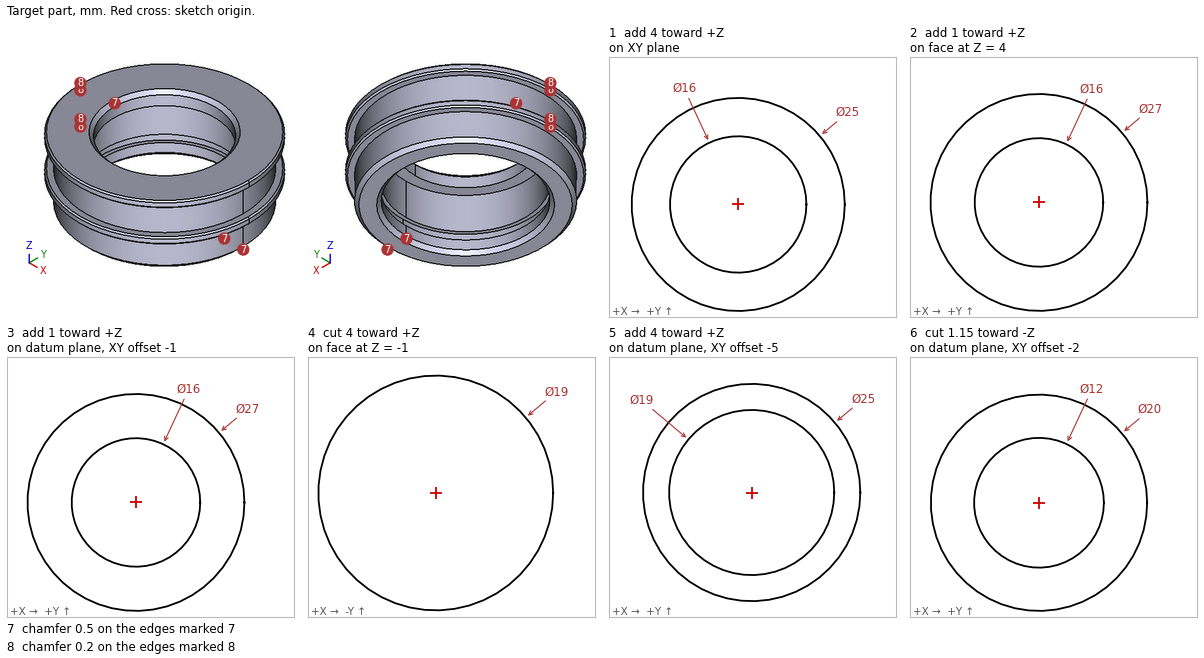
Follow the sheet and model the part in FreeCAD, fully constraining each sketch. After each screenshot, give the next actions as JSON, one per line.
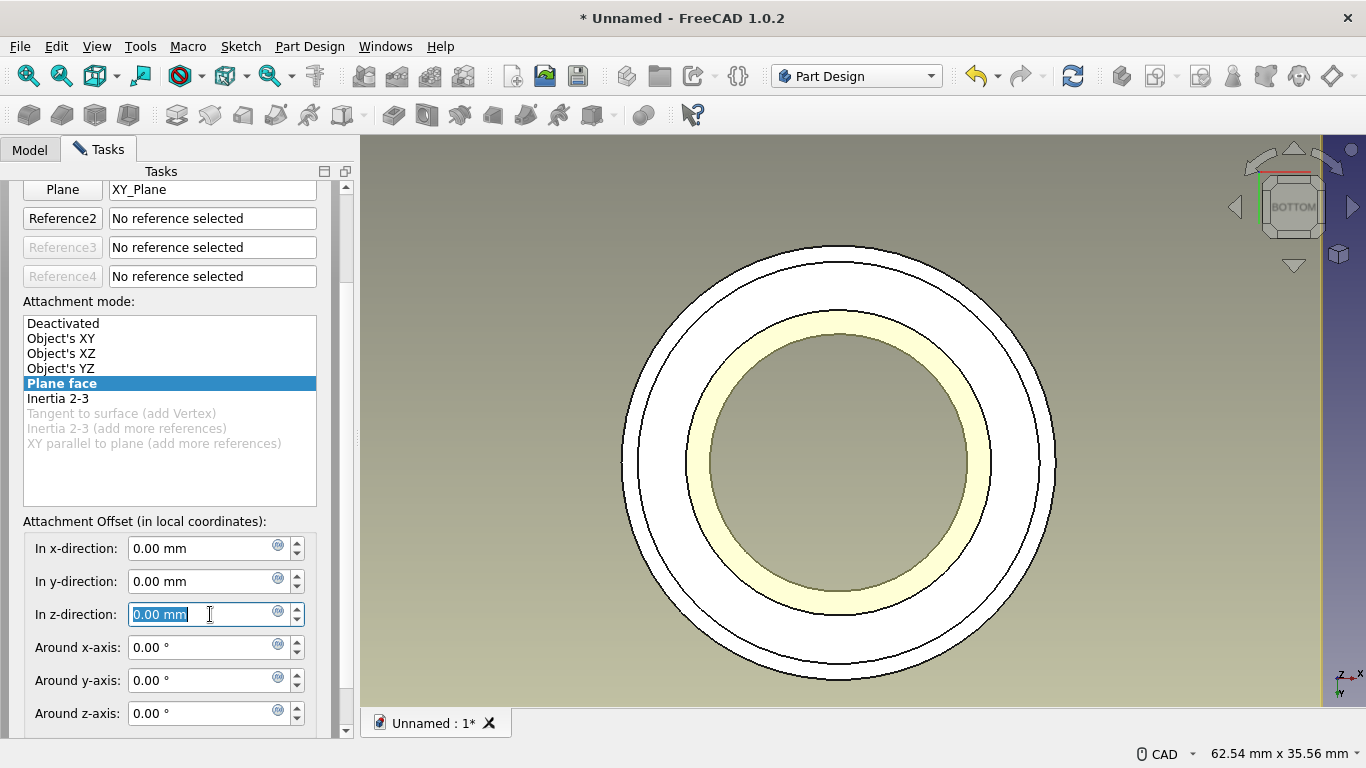
{"action": "type", "text": "-2"}
{"action": "key", "text": "Tab"}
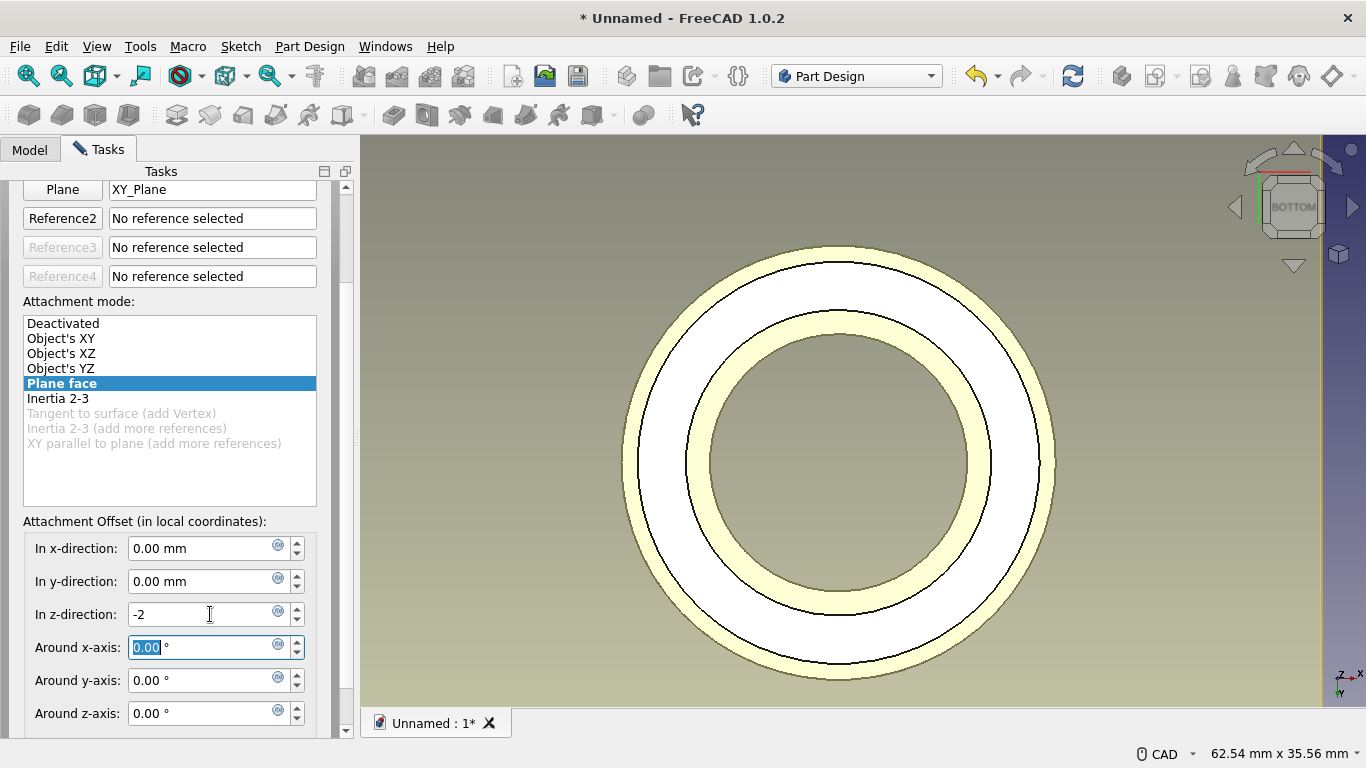
{"action": "scroll", "coordinate": [346, 460], "scroll_direction": "up", "scroll_amount": 3}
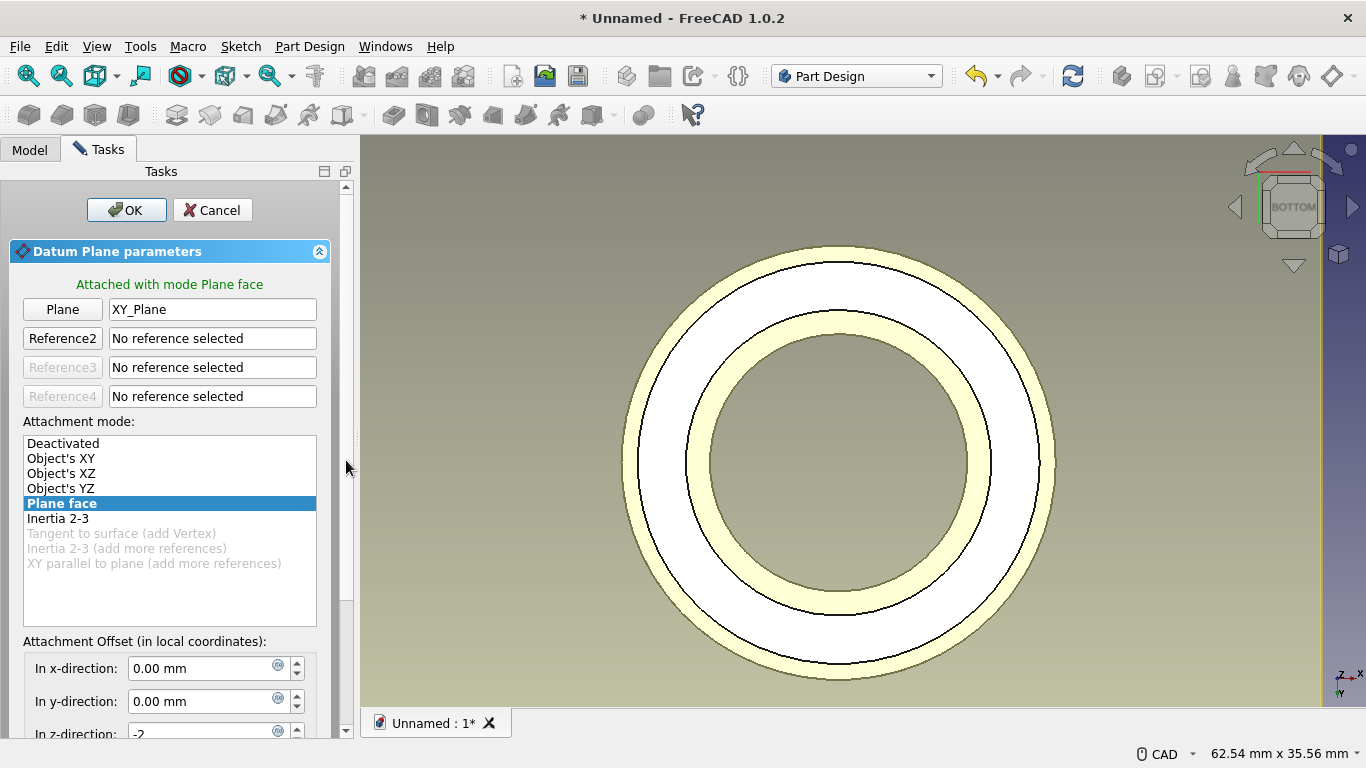
{"action": "left_click", "coordinate": [127, 210]}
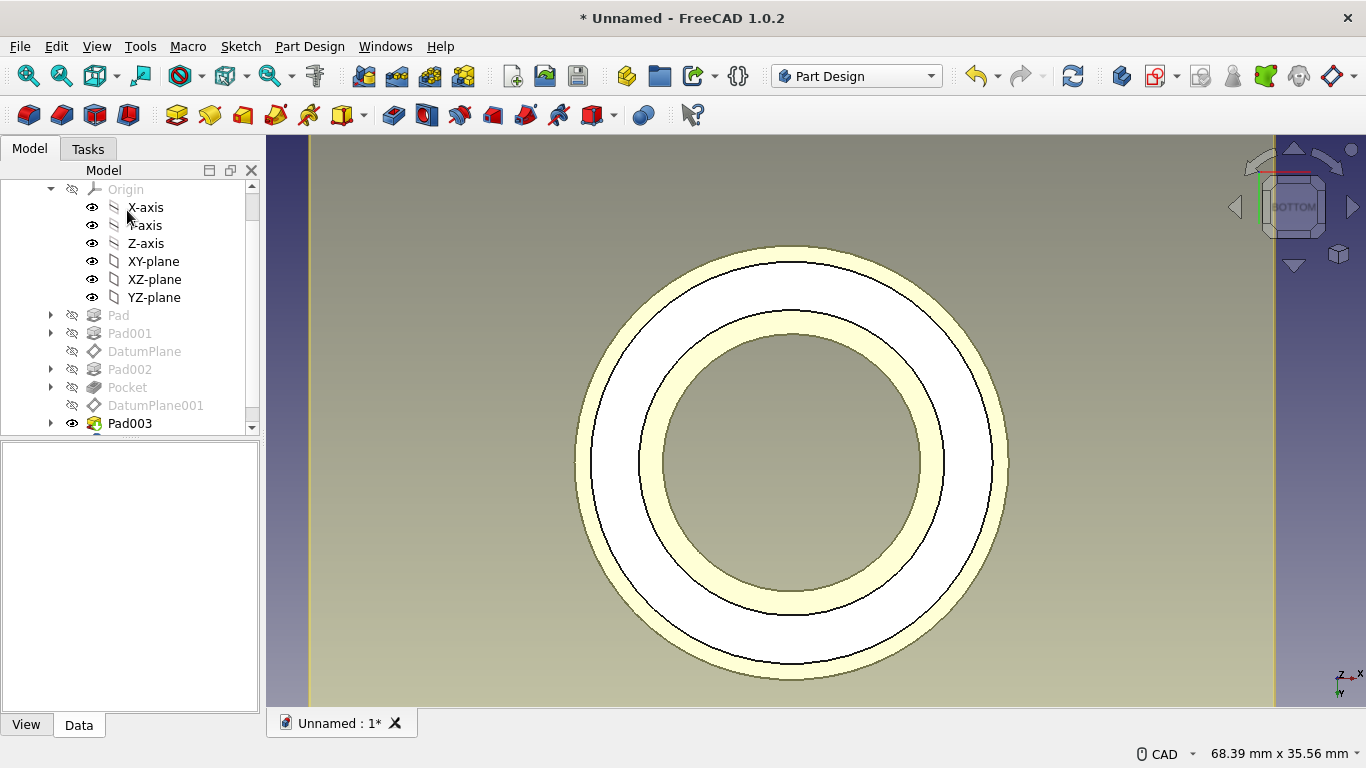
{"action": "scroll", "coordinate": [141, 311], "scroll_direction": "down", "scroll_amount": 3}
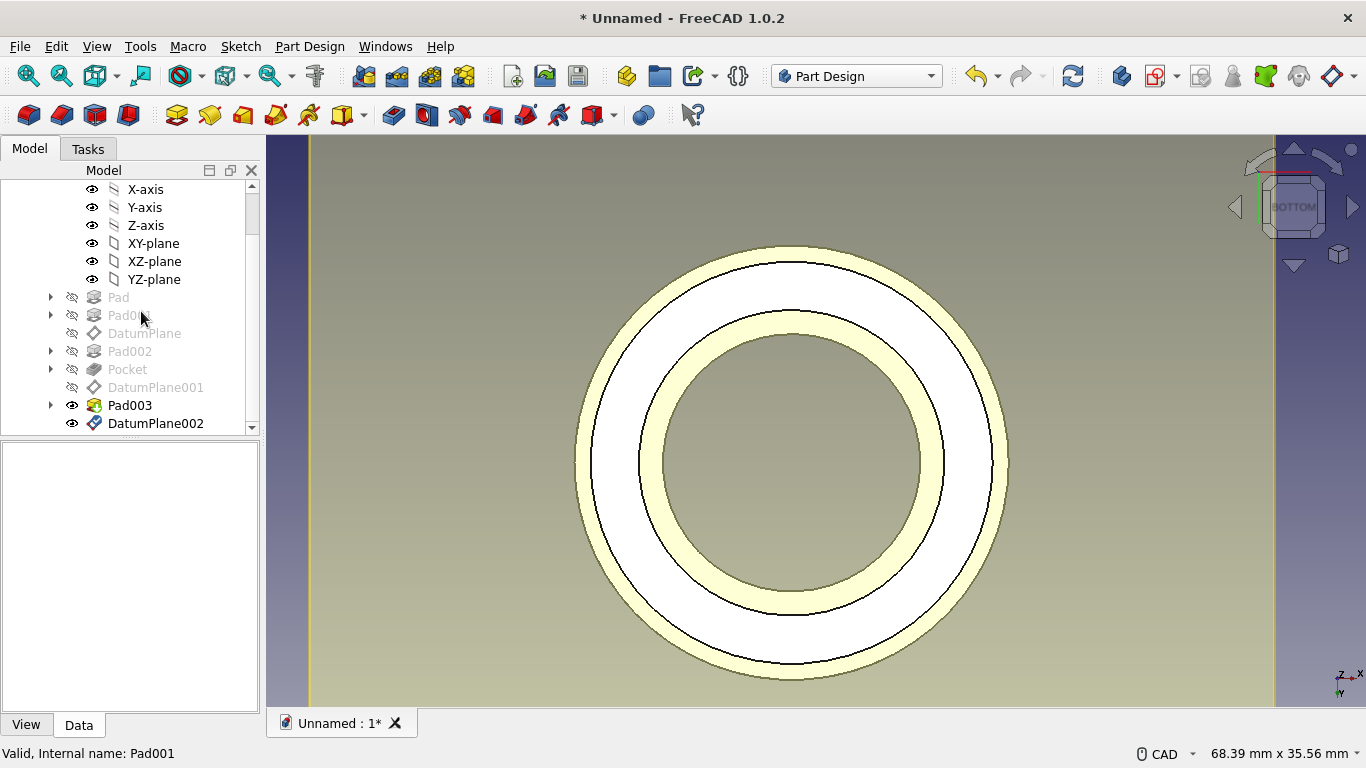
{"action": "left_click", "coordinate": [117, 423]}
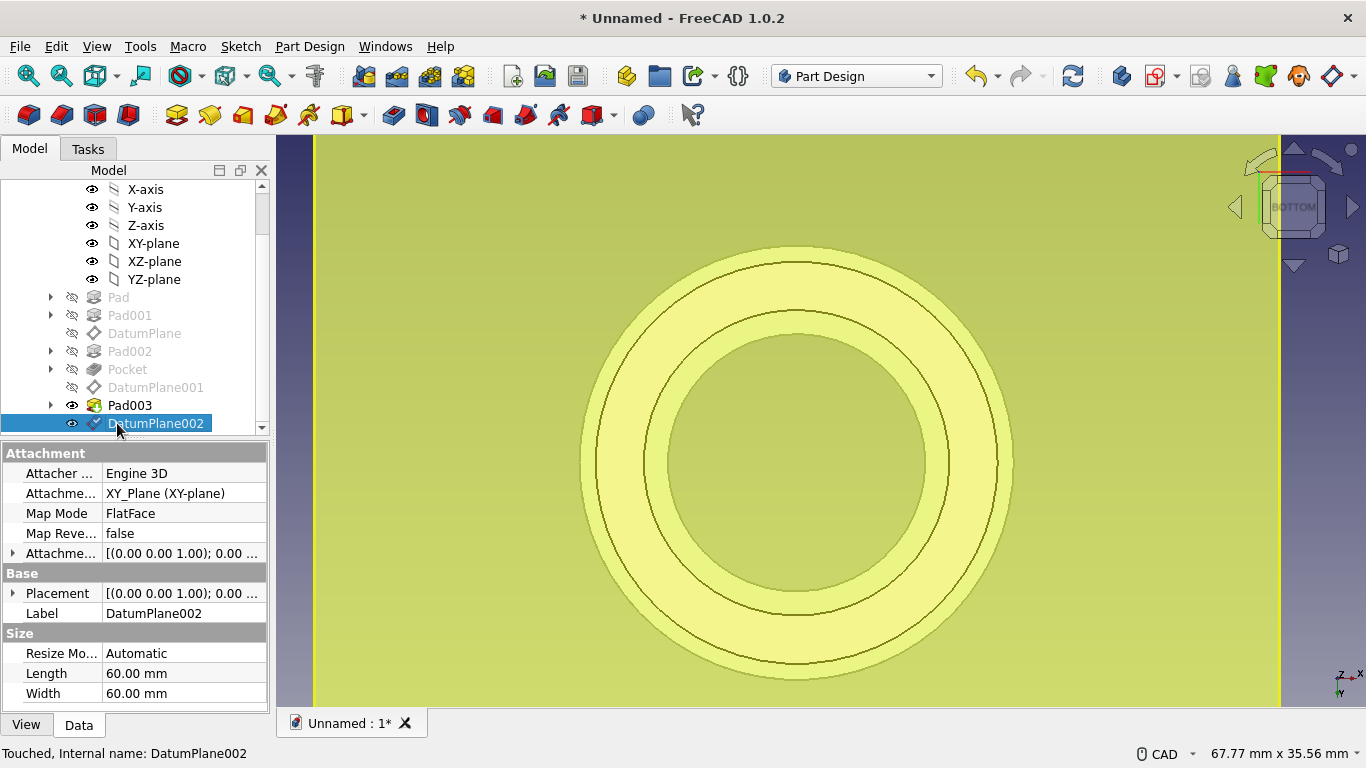
{"action": "left_click", "coordinate": [1154, 76]}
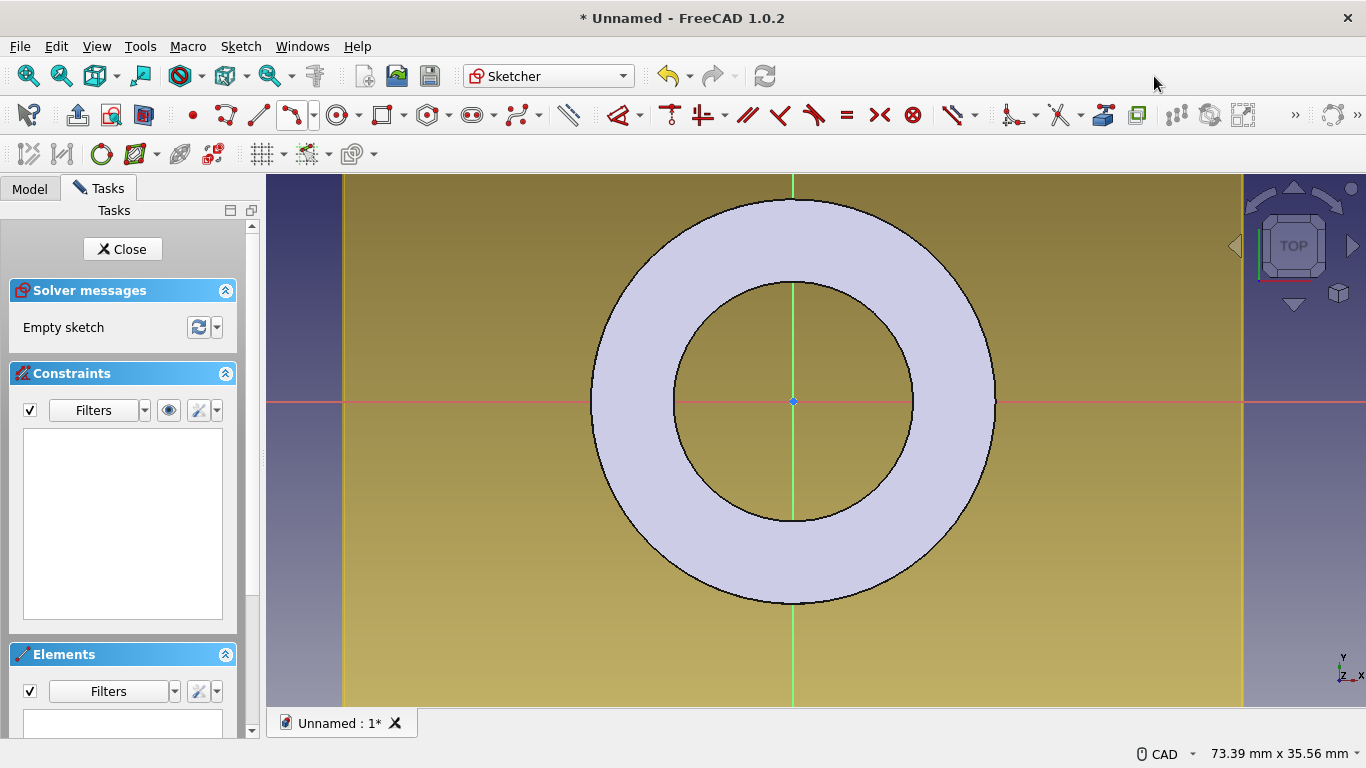
{"action": "left_click", "coordinate": [144, 116]}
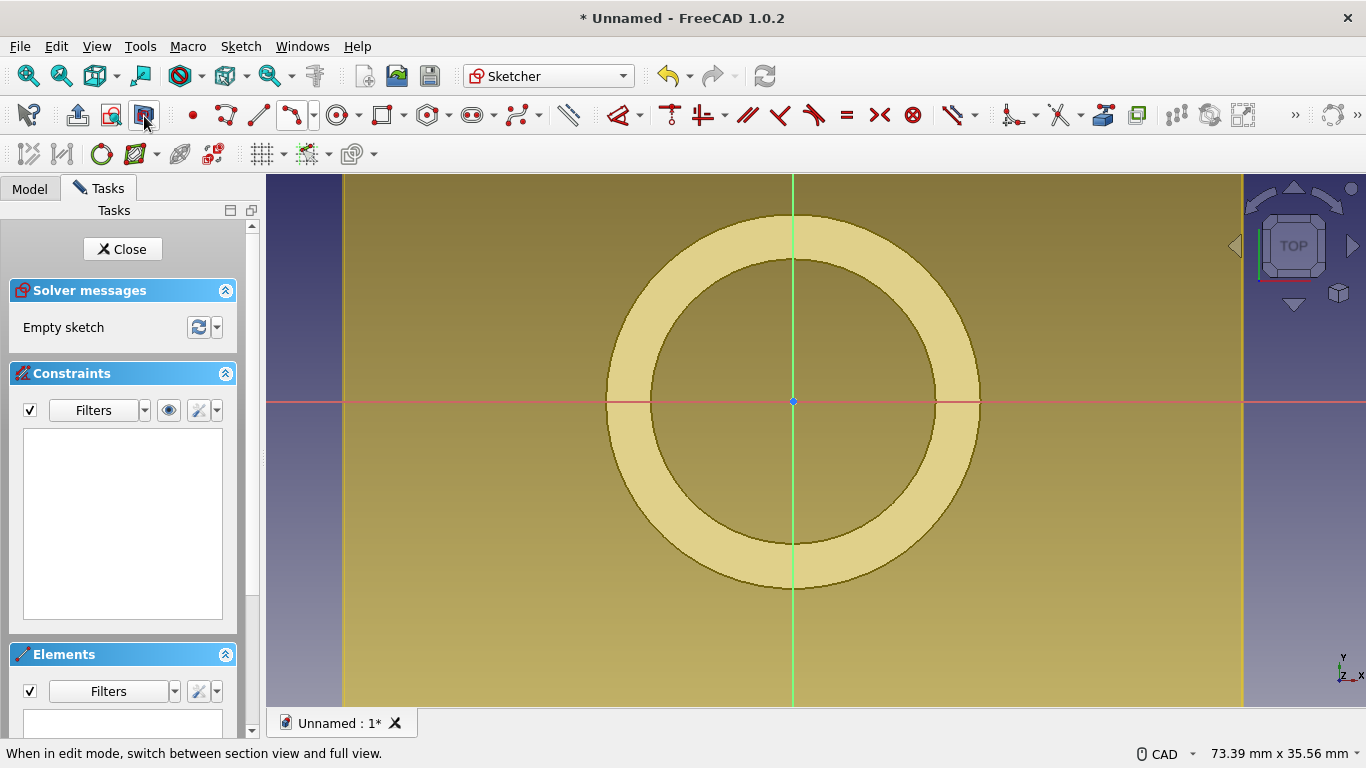
{"action": "left_click", "coordinate": [336, 116]}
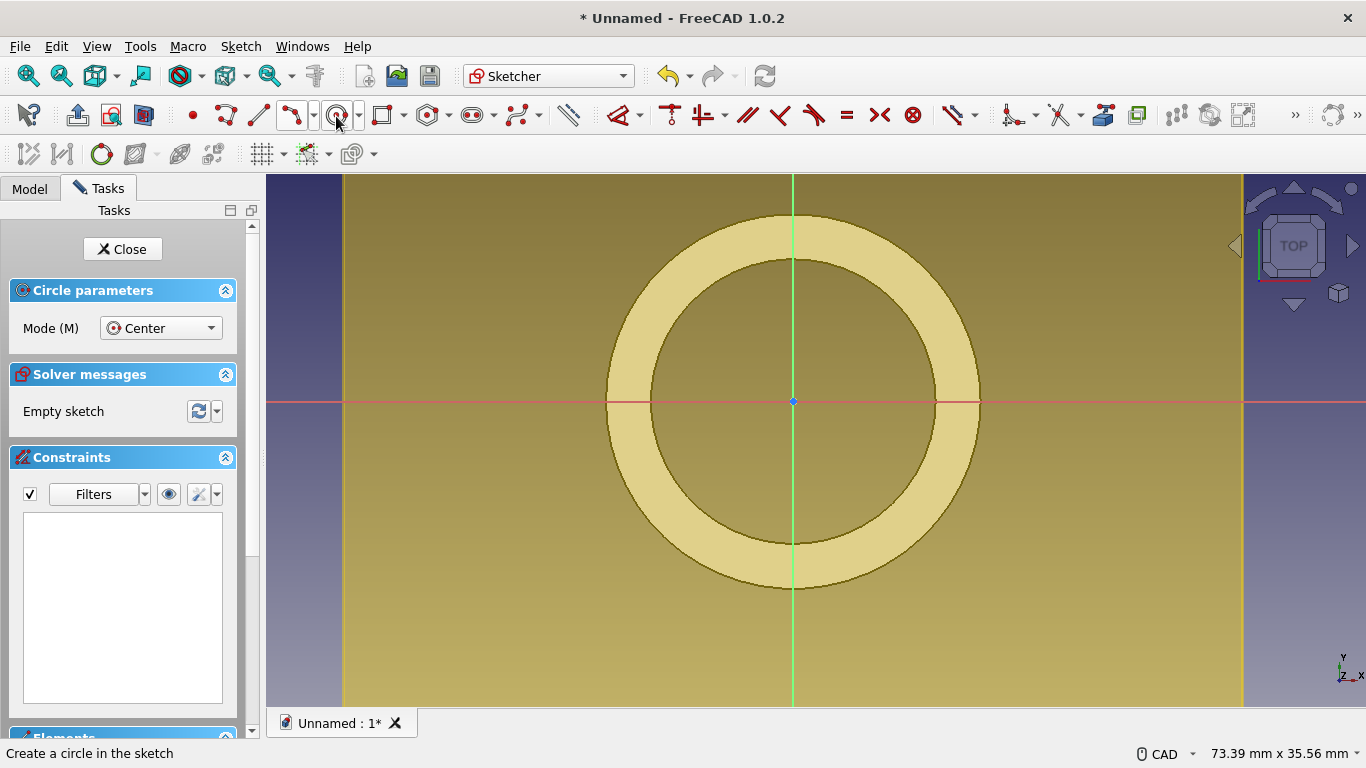
{"action": "left_click", "coordinate": [793, 402]}
{"action": "left_click", "coordinate": [899, 296]}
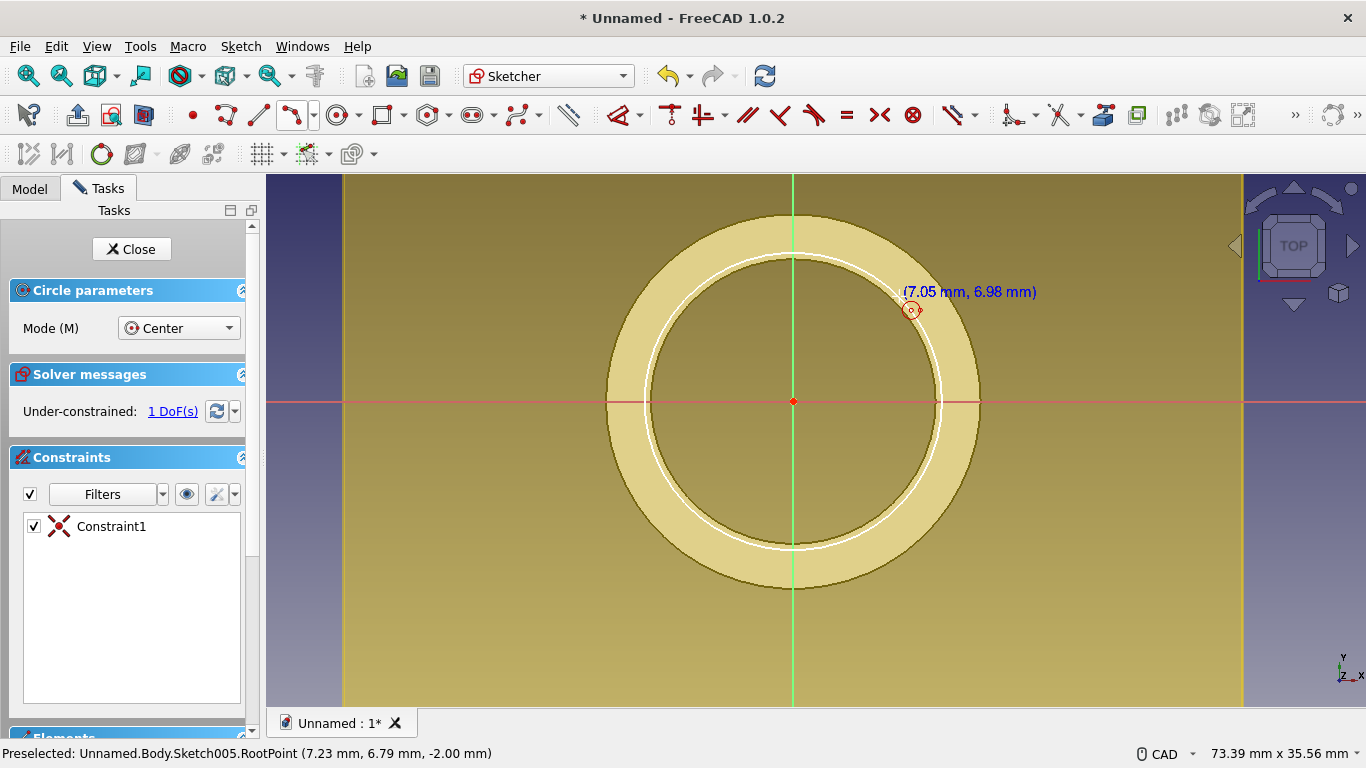
{"action": "left_click", "coordinate": [793, 402]}
{"action": "left_click", "coordinate": [857, 338]}
{"action": "key", "text": "Escape"}